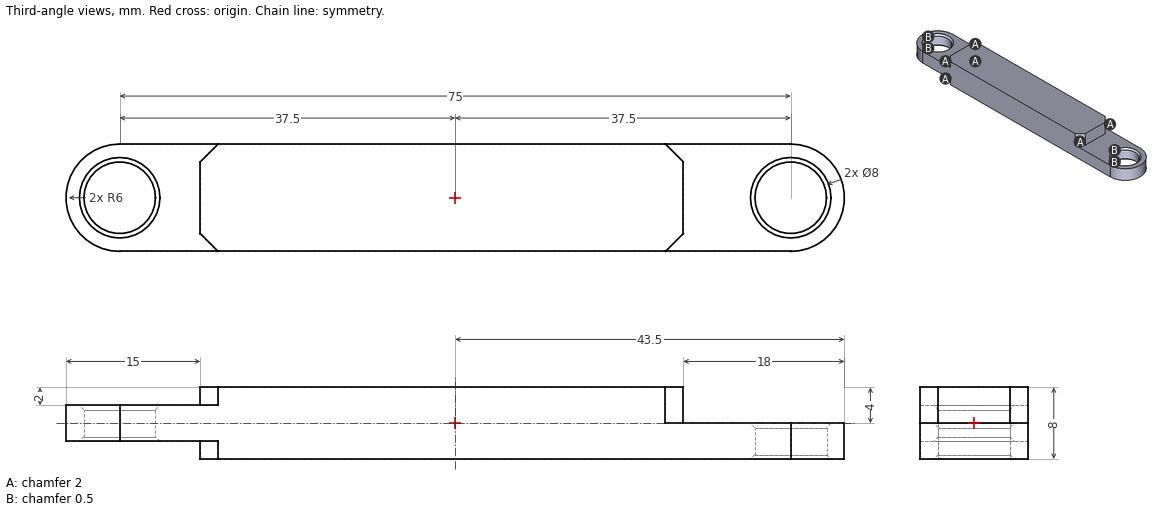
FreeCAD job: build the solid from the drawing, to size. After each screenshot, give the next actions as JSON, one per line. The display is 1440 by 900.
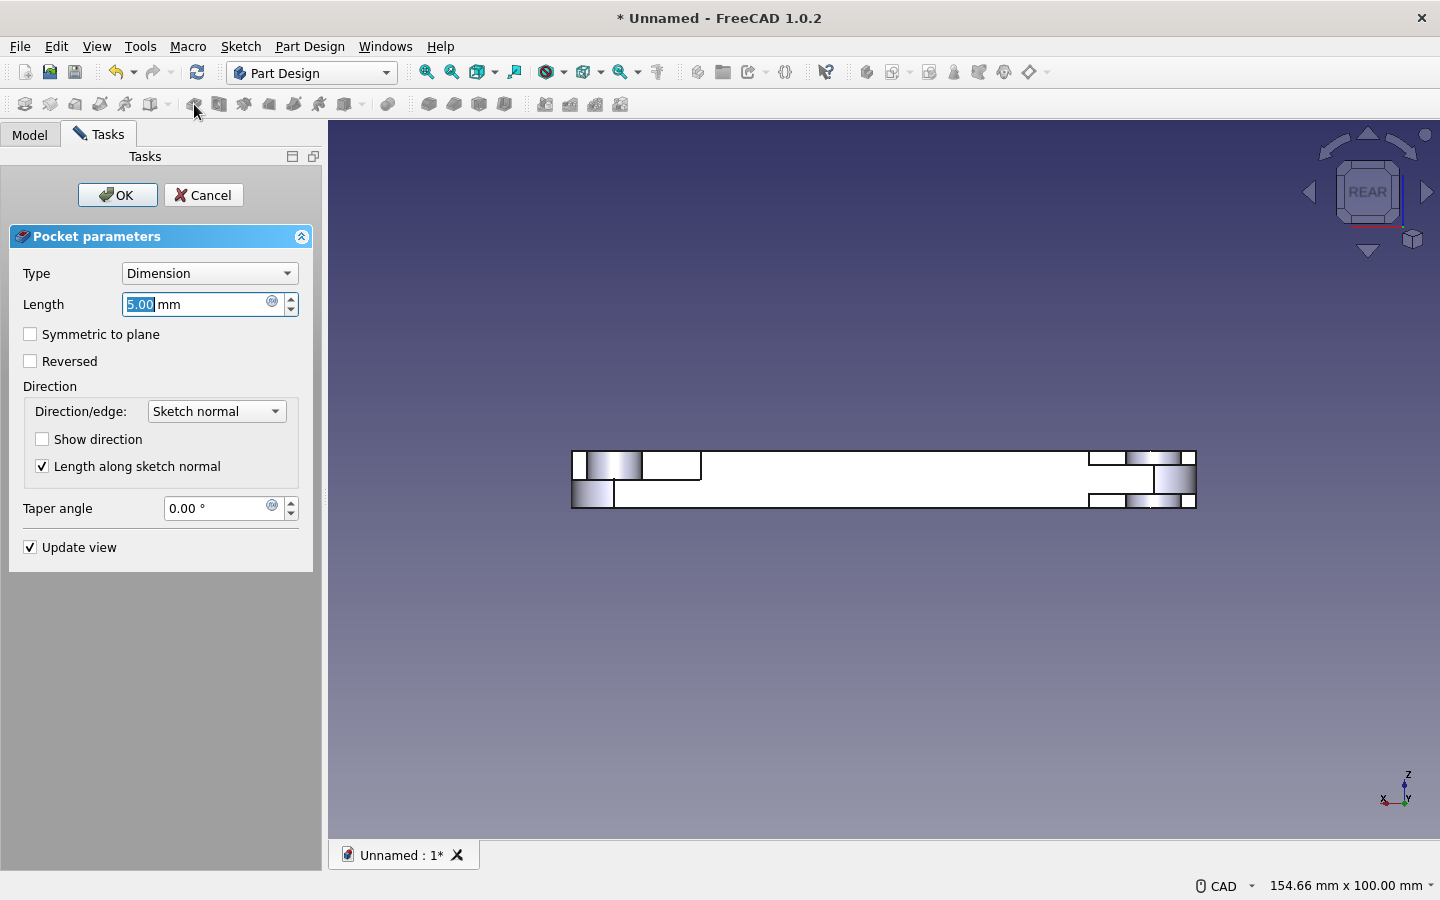
{"action": "left_click", "coordinate": [210, 274]}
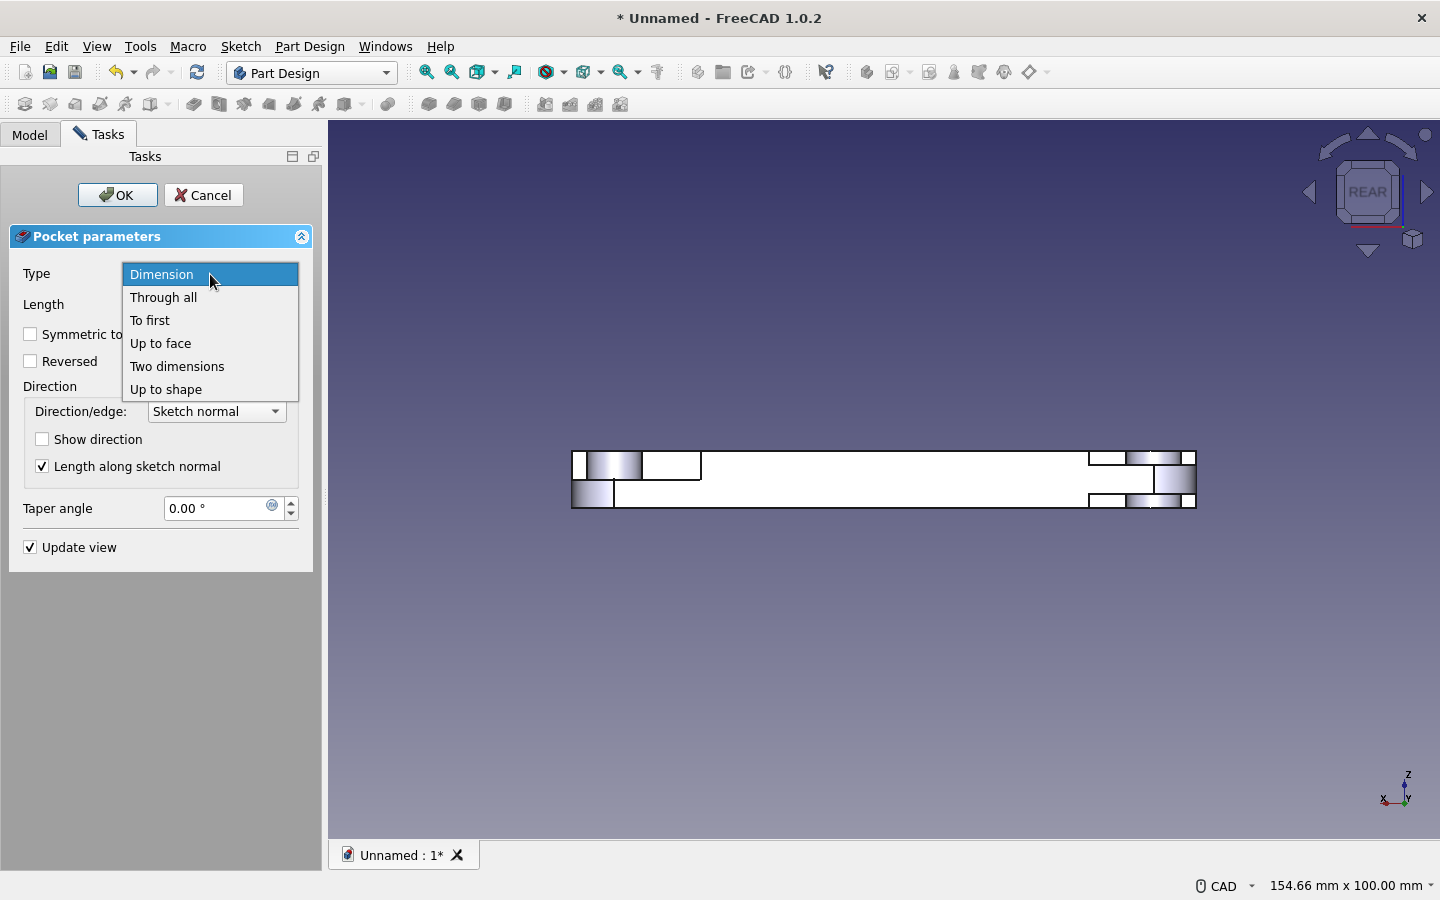
{"action": "left_click", "coordinate": [208, 298]}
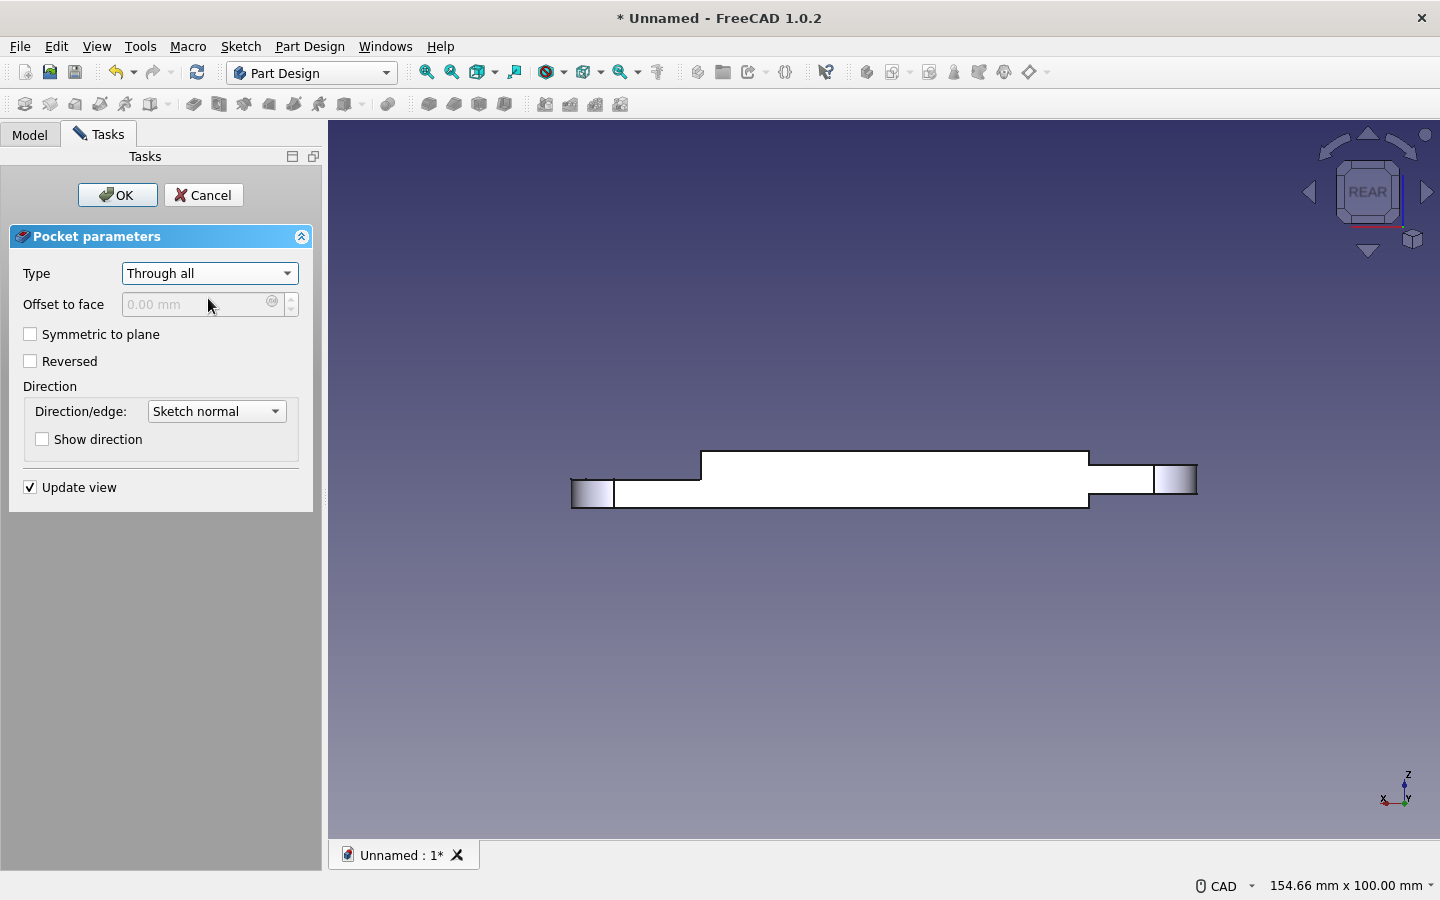
{"action": "left_click", "coordinate": [118, 195]}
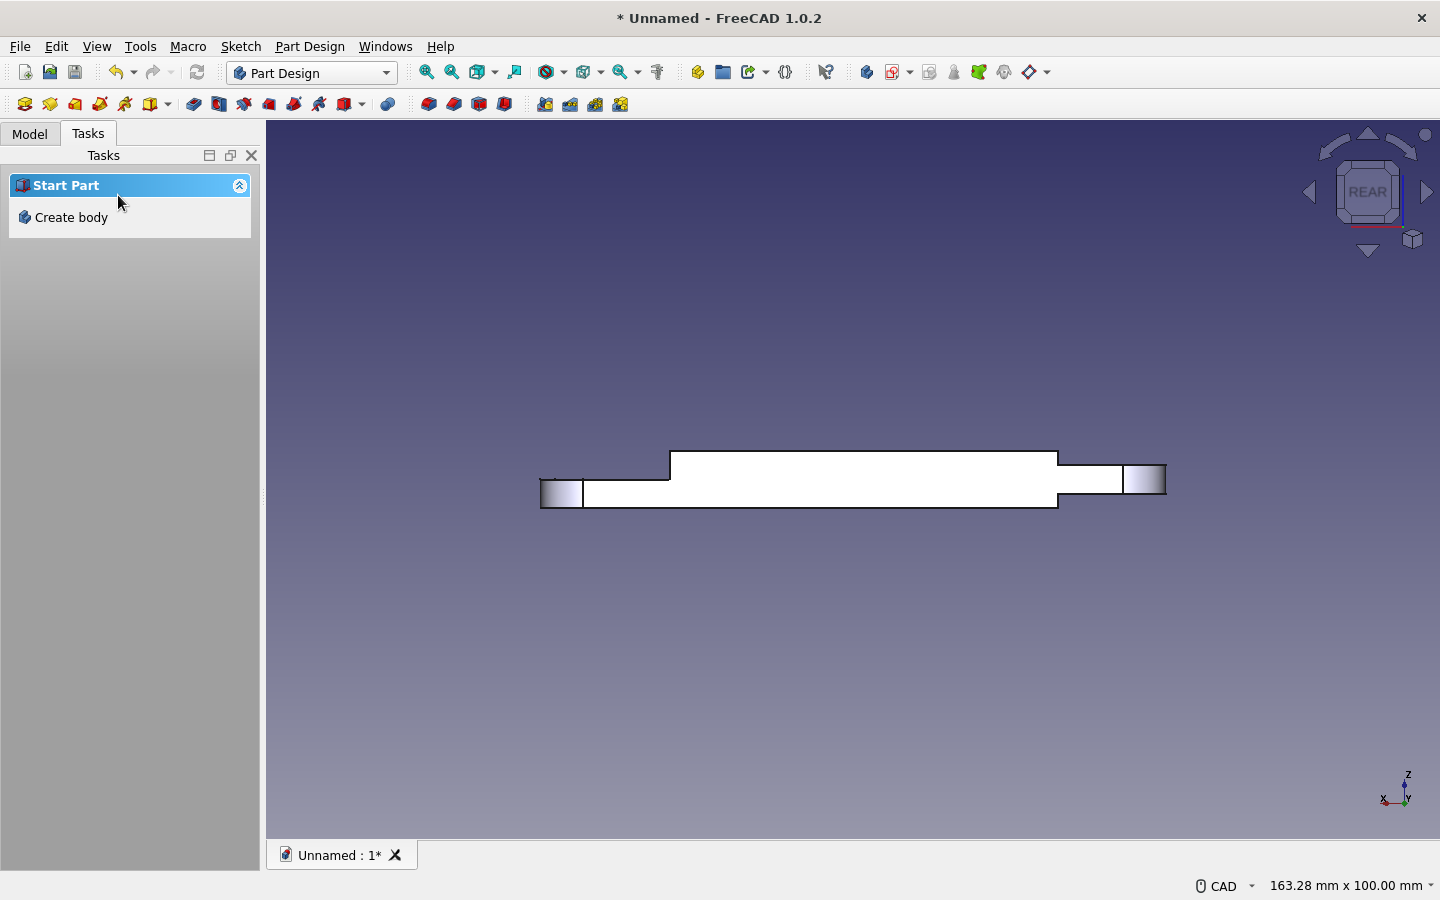
{"action": "left_click", "coordinate": [1058, 457]}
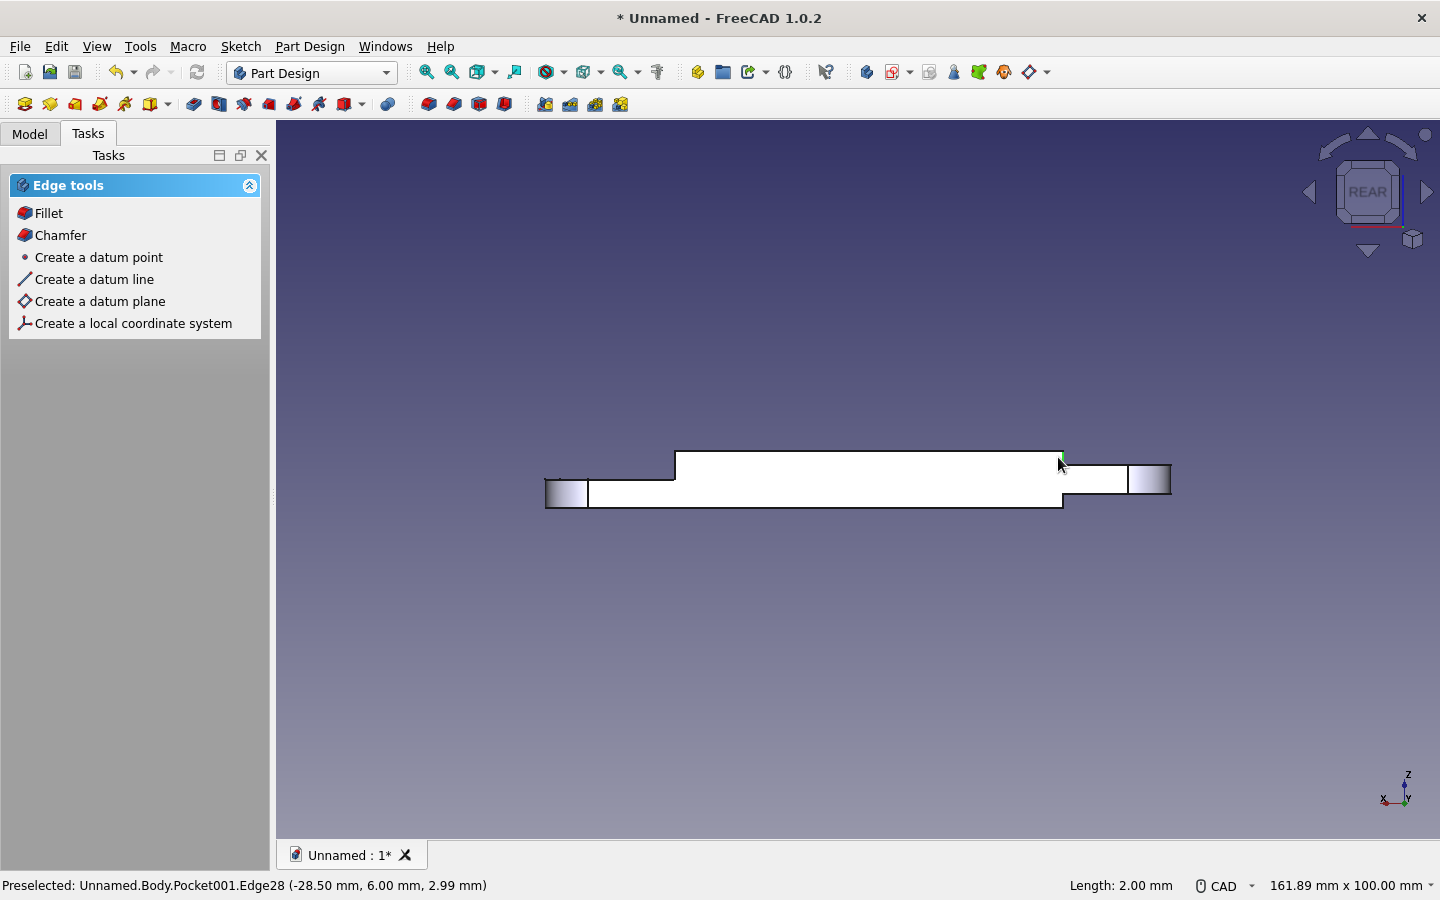
{"action": "left_click", "coordinate": [1063, 500], "text": "ctrl"}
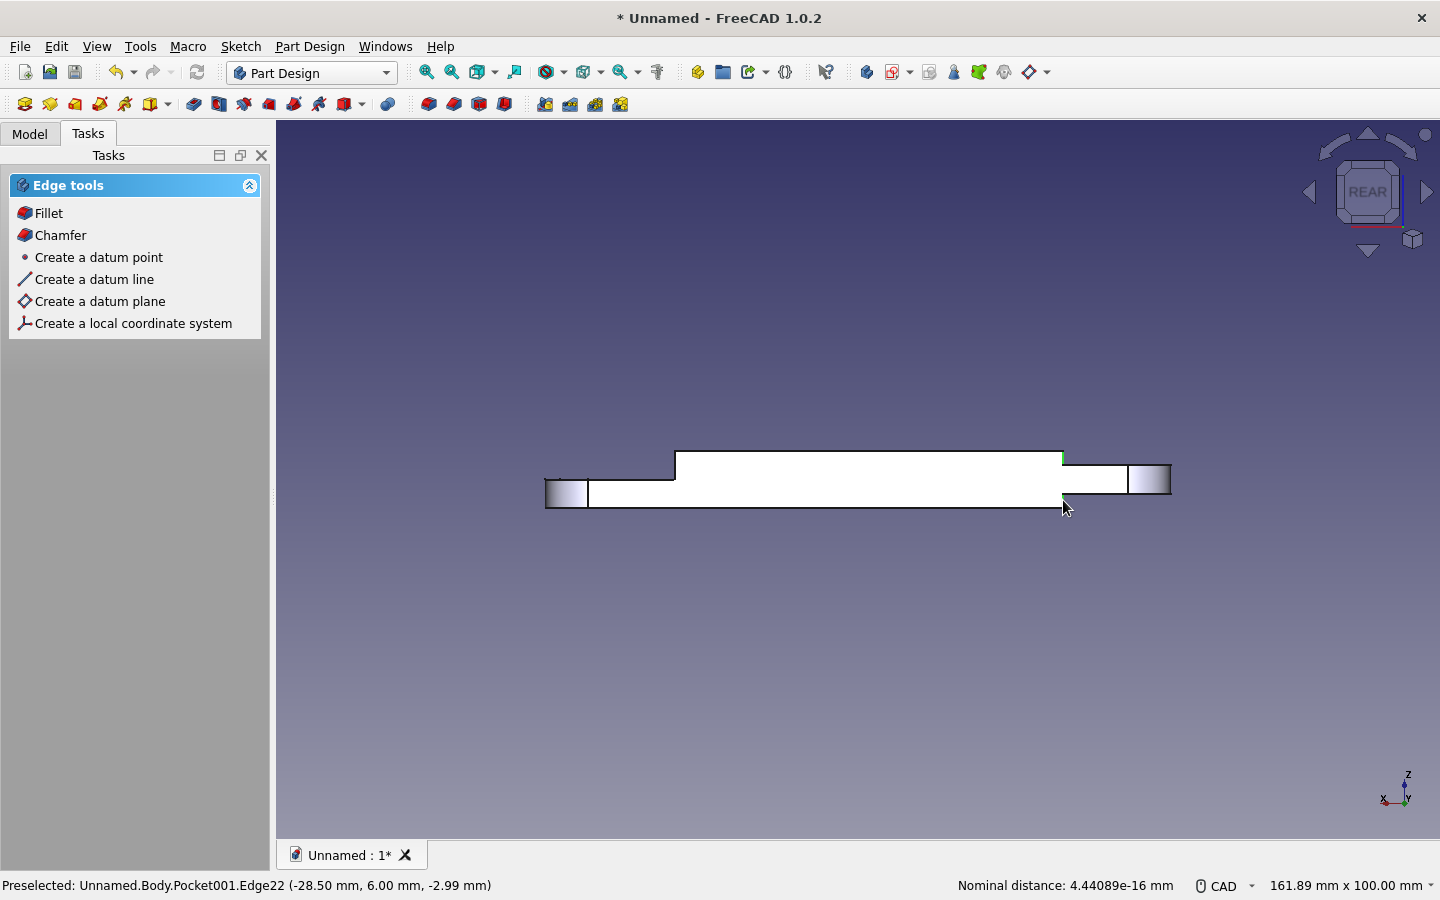
{"action": "key", "text": "0"}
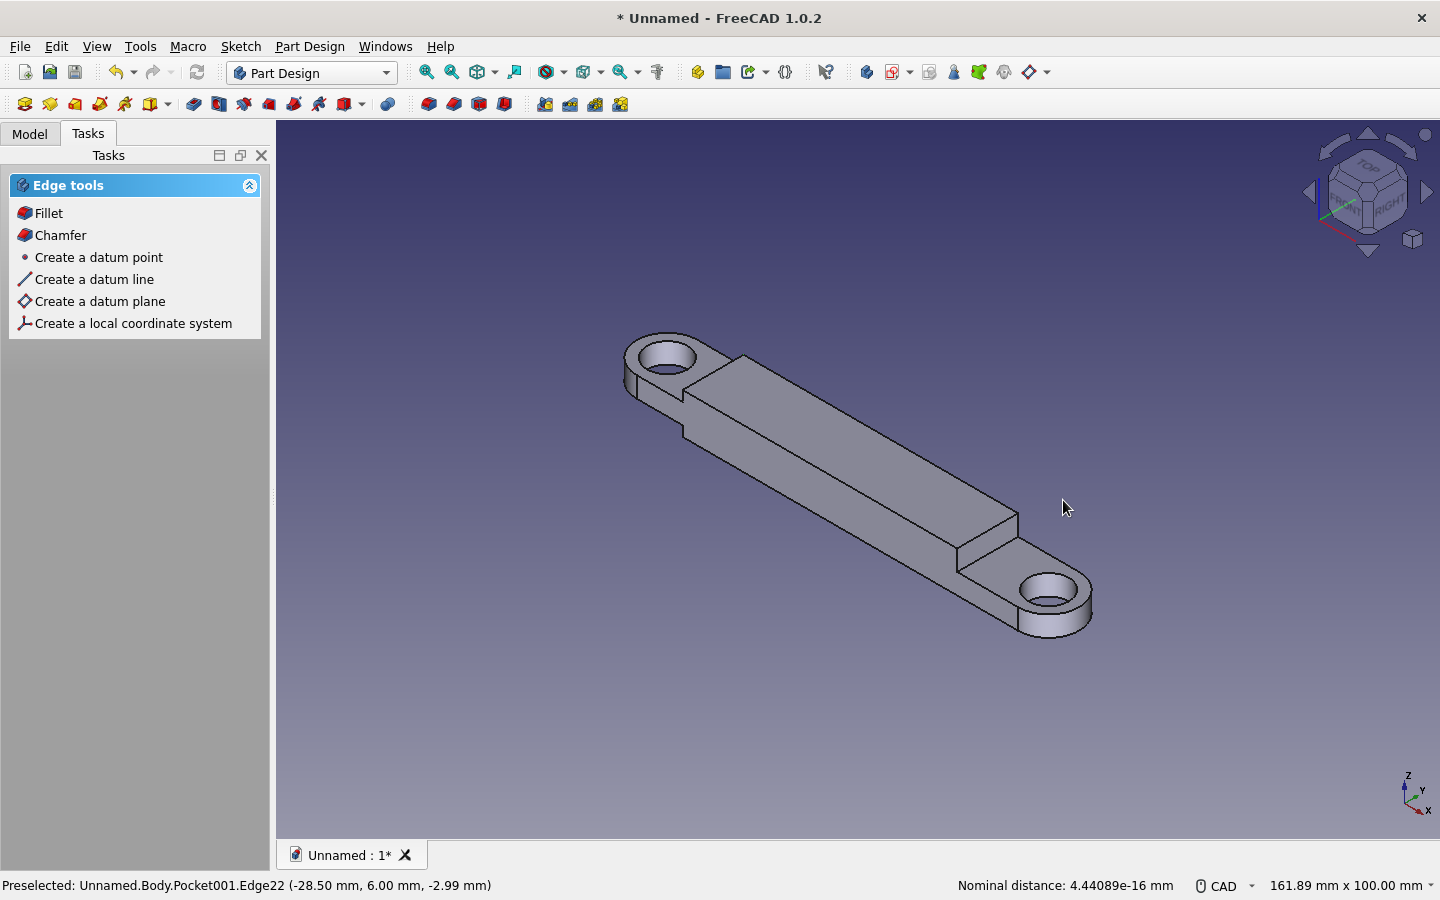
{"action": "left_click", "coordinate": [957, 559], "text": "ctrl"}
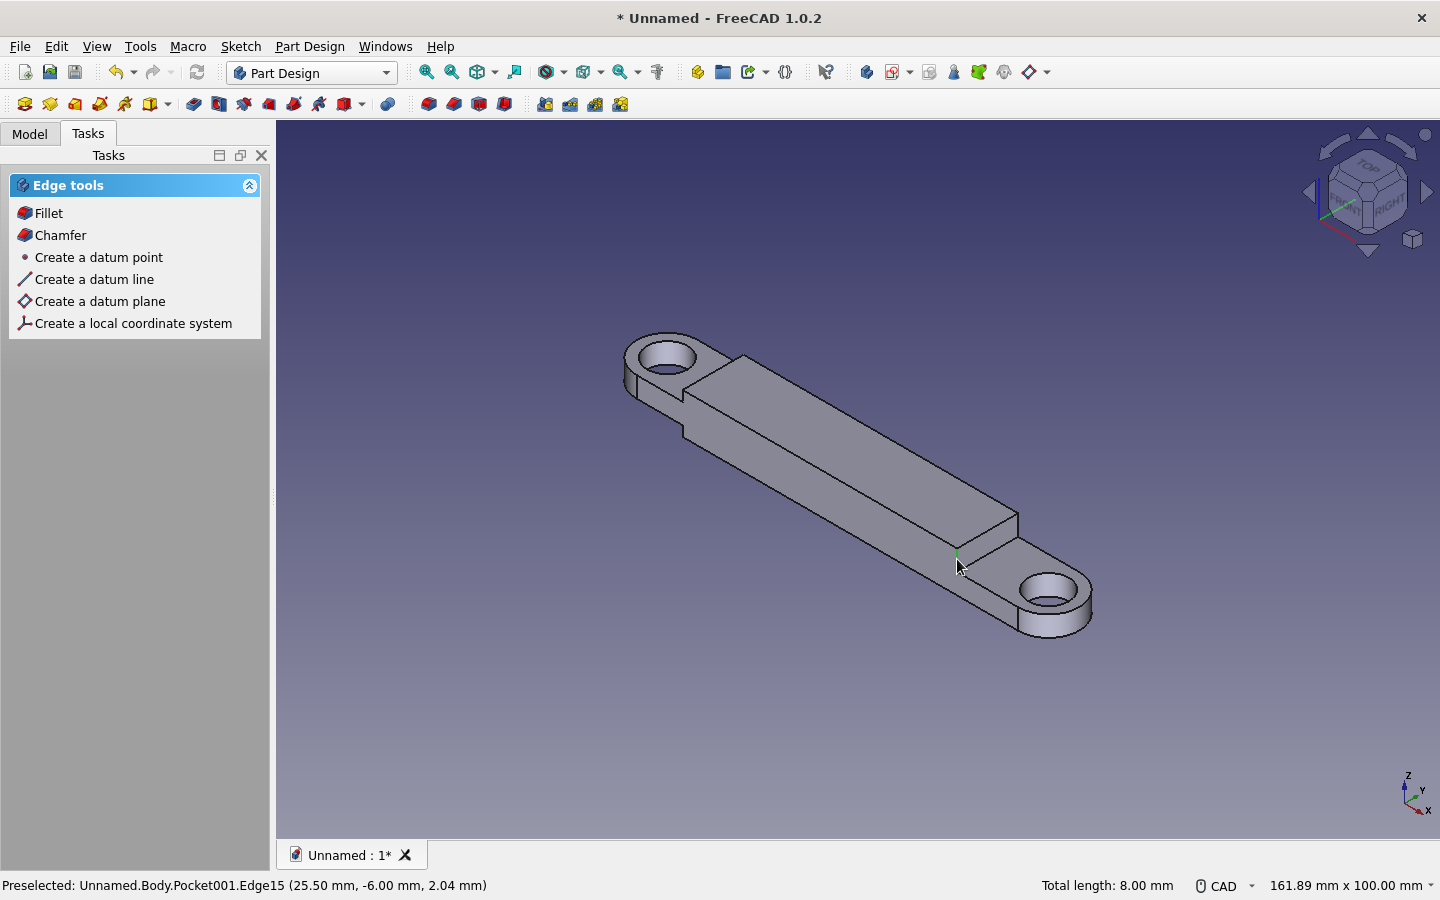
{"action": "key", "text": "2"}